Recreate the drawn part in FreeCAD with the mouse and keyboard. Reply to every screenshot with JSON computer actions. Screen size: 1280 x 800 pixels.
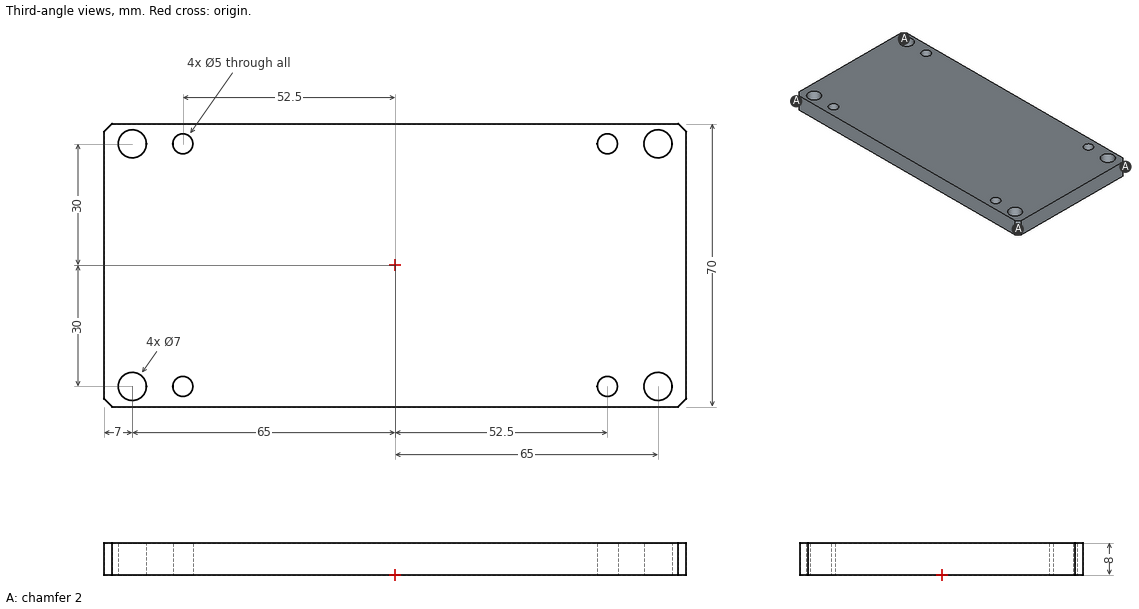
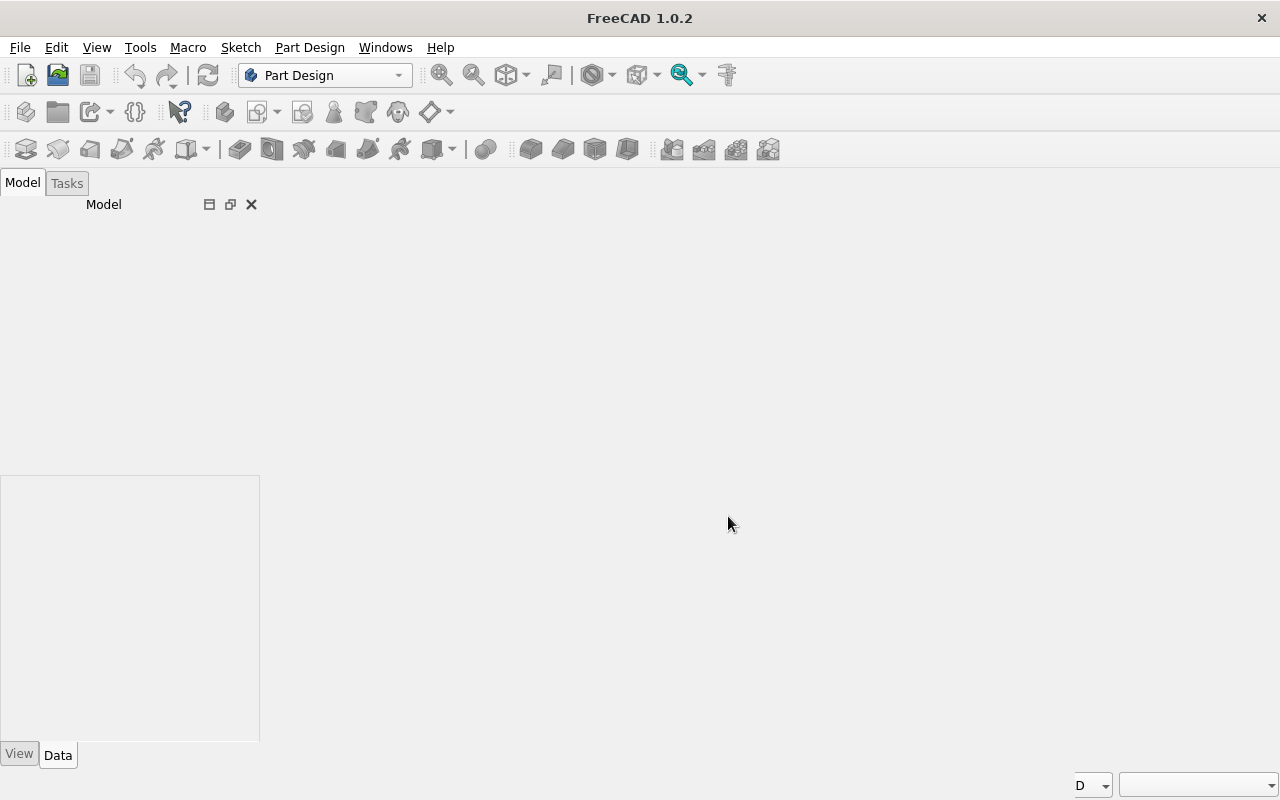
{"action": "left_click", "coordinate": [26, 76]}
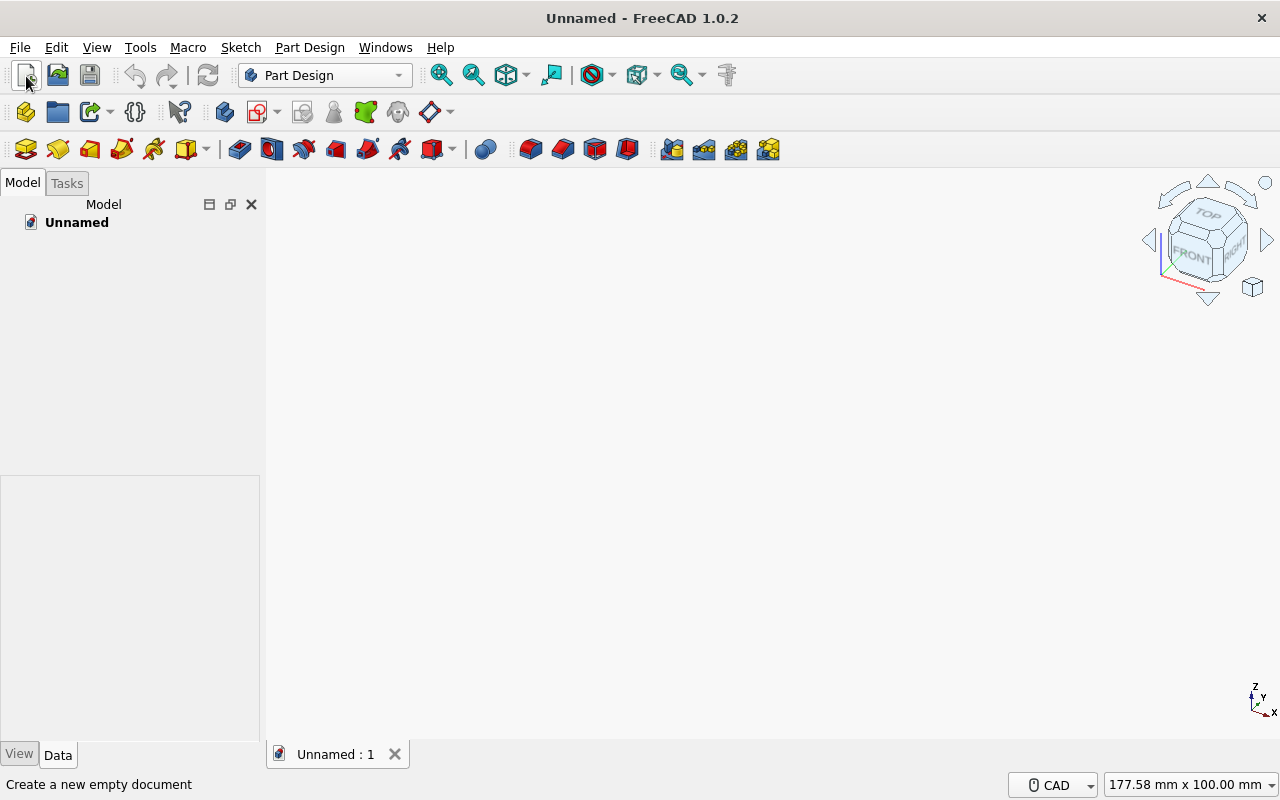
{"action": "left_click", "coordinate": [258, 112]}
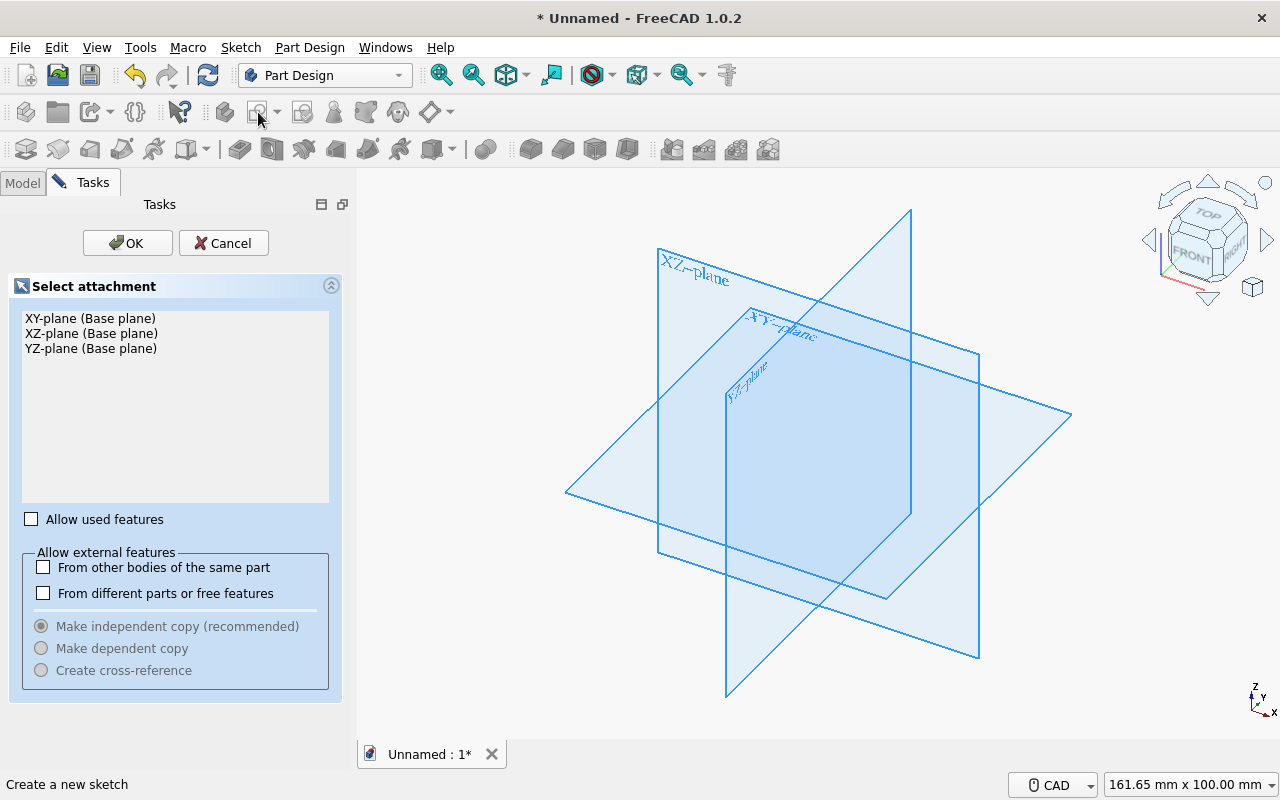
{"action": "left_click", "coordinate": [82, 318]}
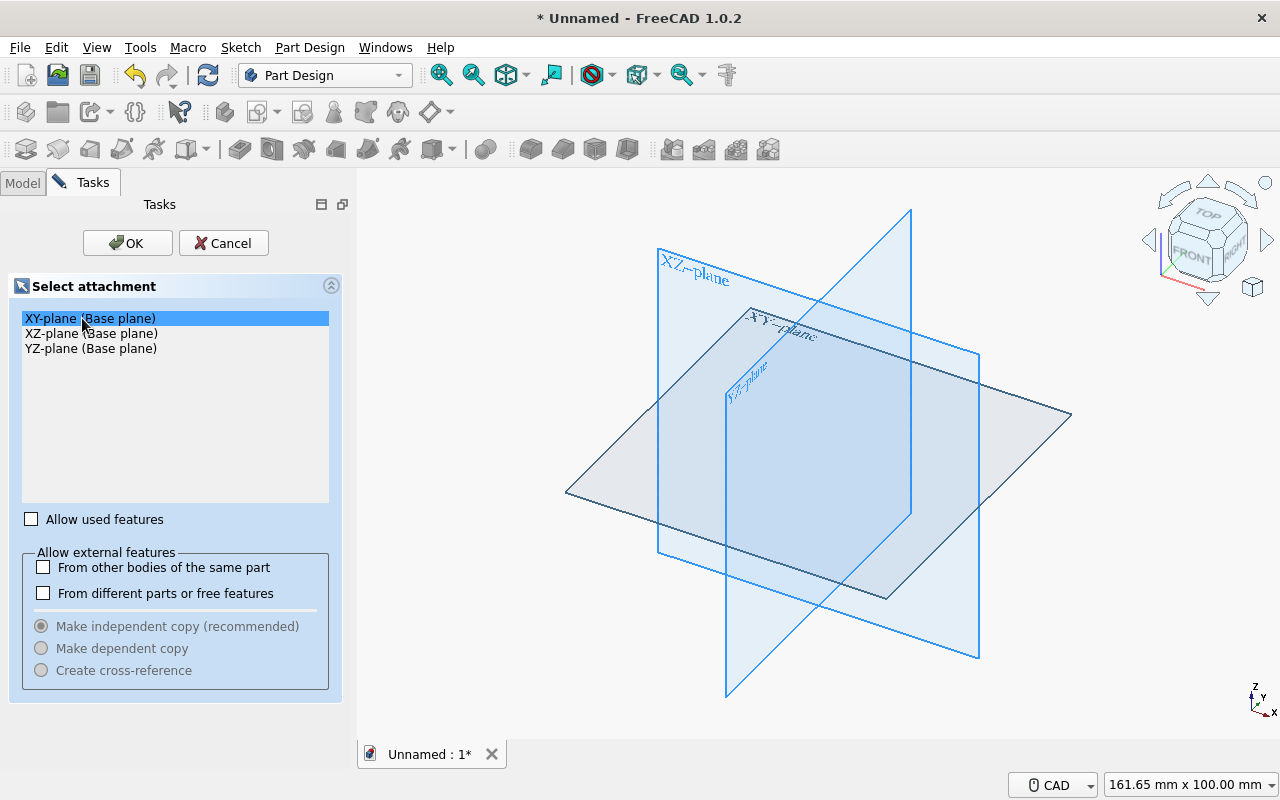
{"action": "left_click", "coordinate": [128, 243]}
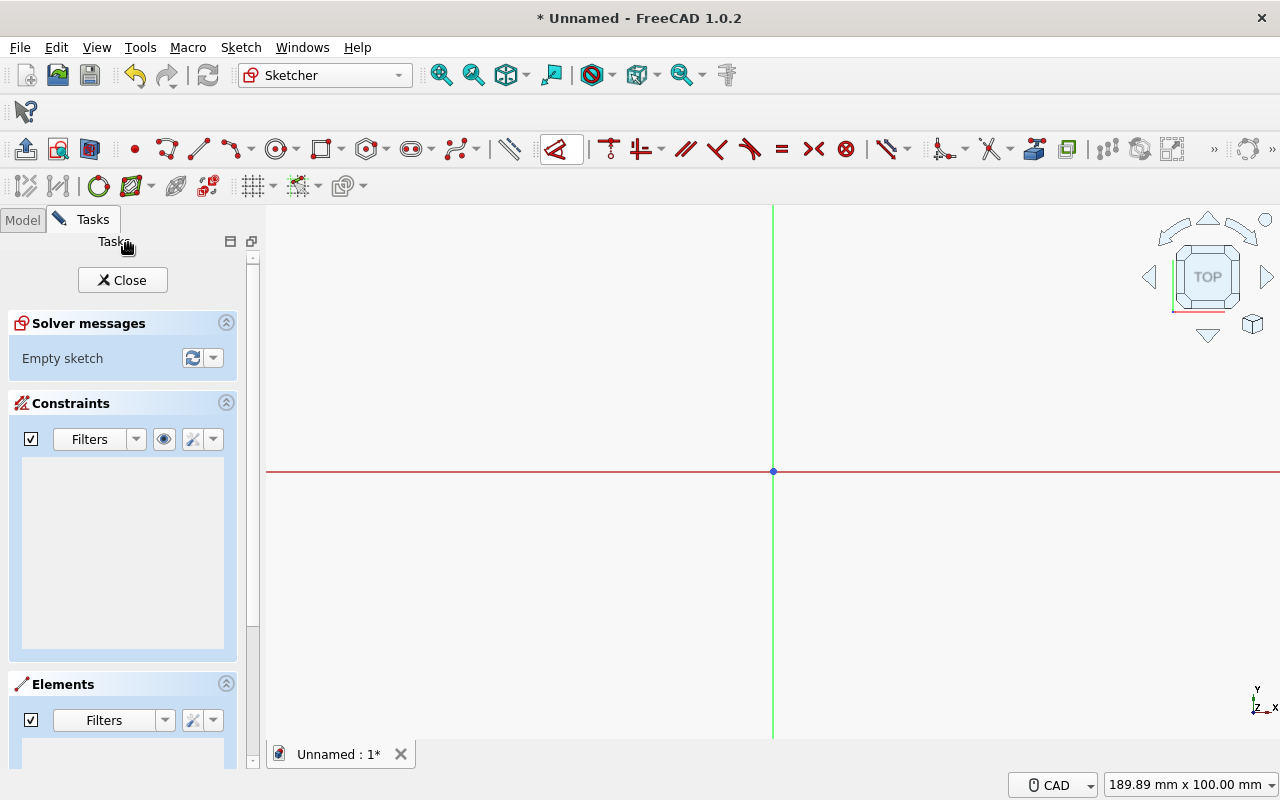
{"action": "scroll", "coordinate": [395, 472], "scroll_direction": "down", "scroll_amount": 1}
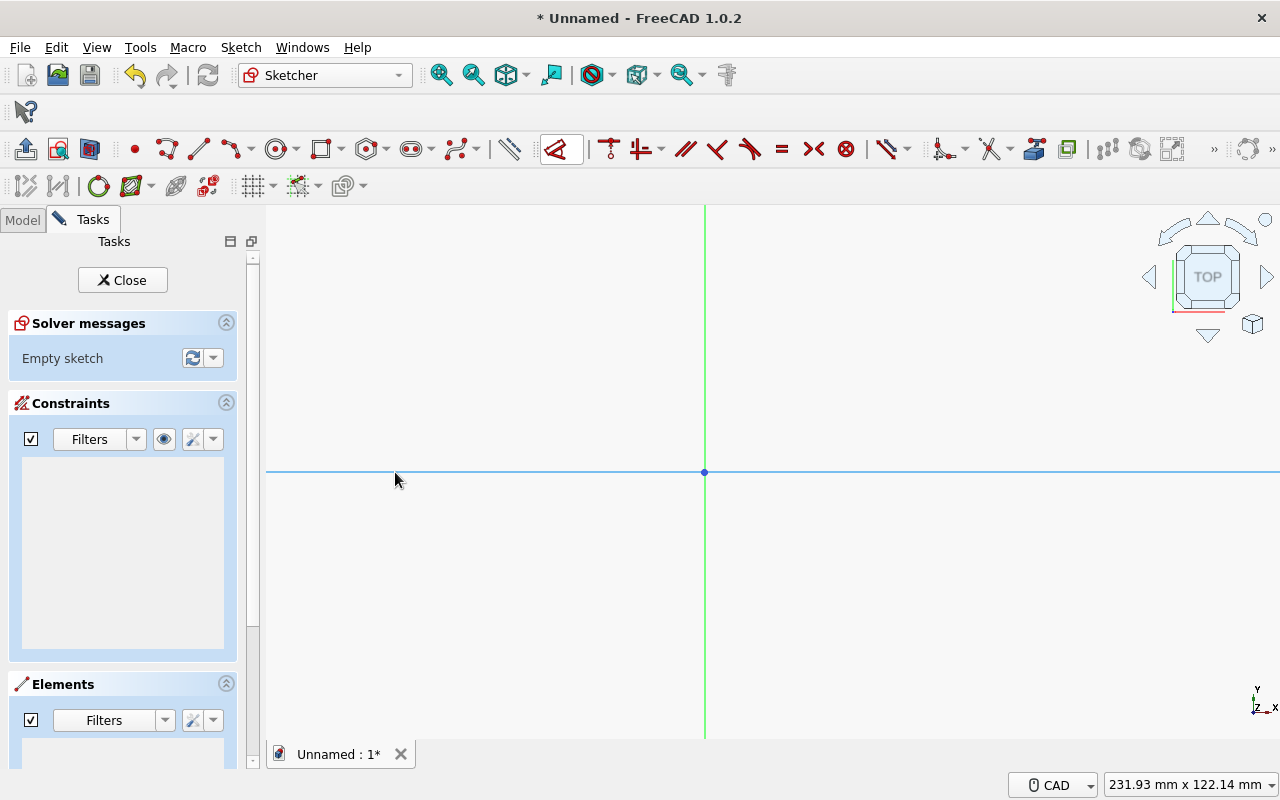
{"action": "key", "text": "g v"}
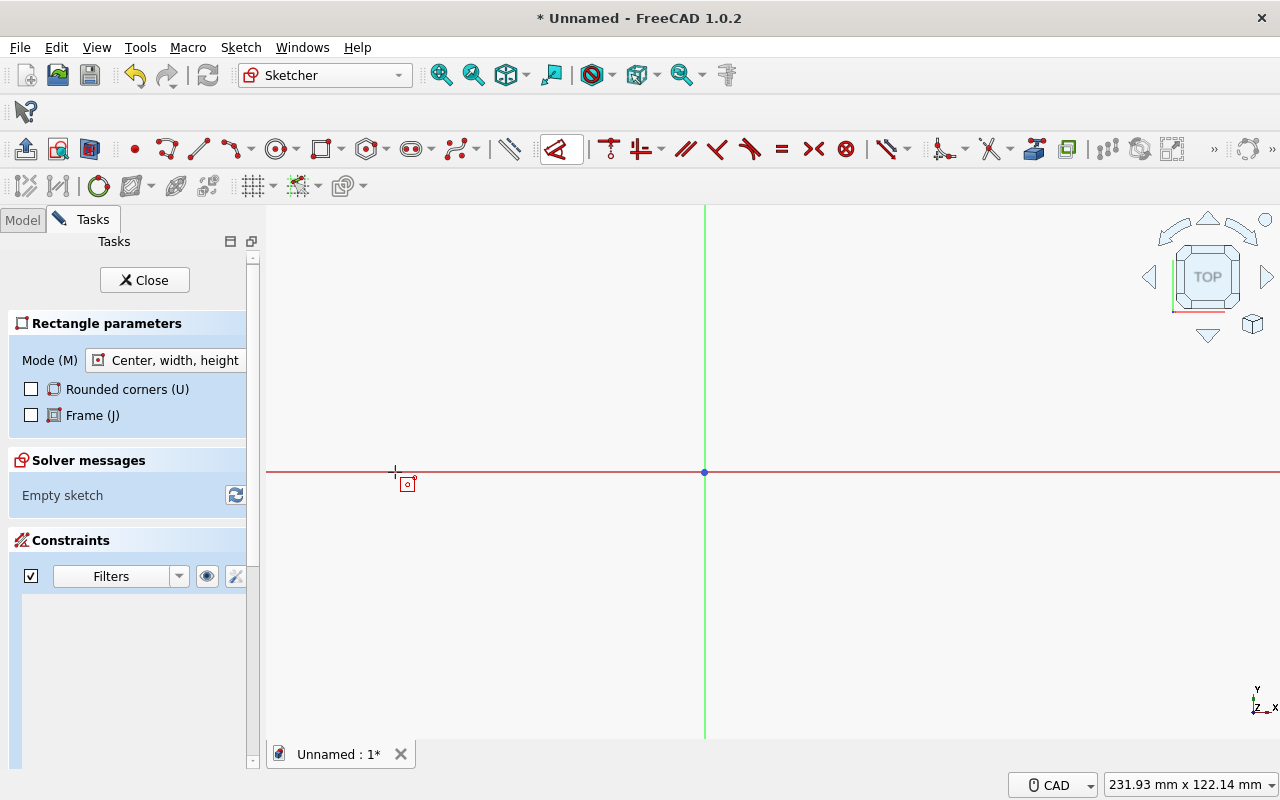
{"action": "left_click", "coordinate": [705, 472]}
{"action": "left_click", "coordinate": [1019, 319]}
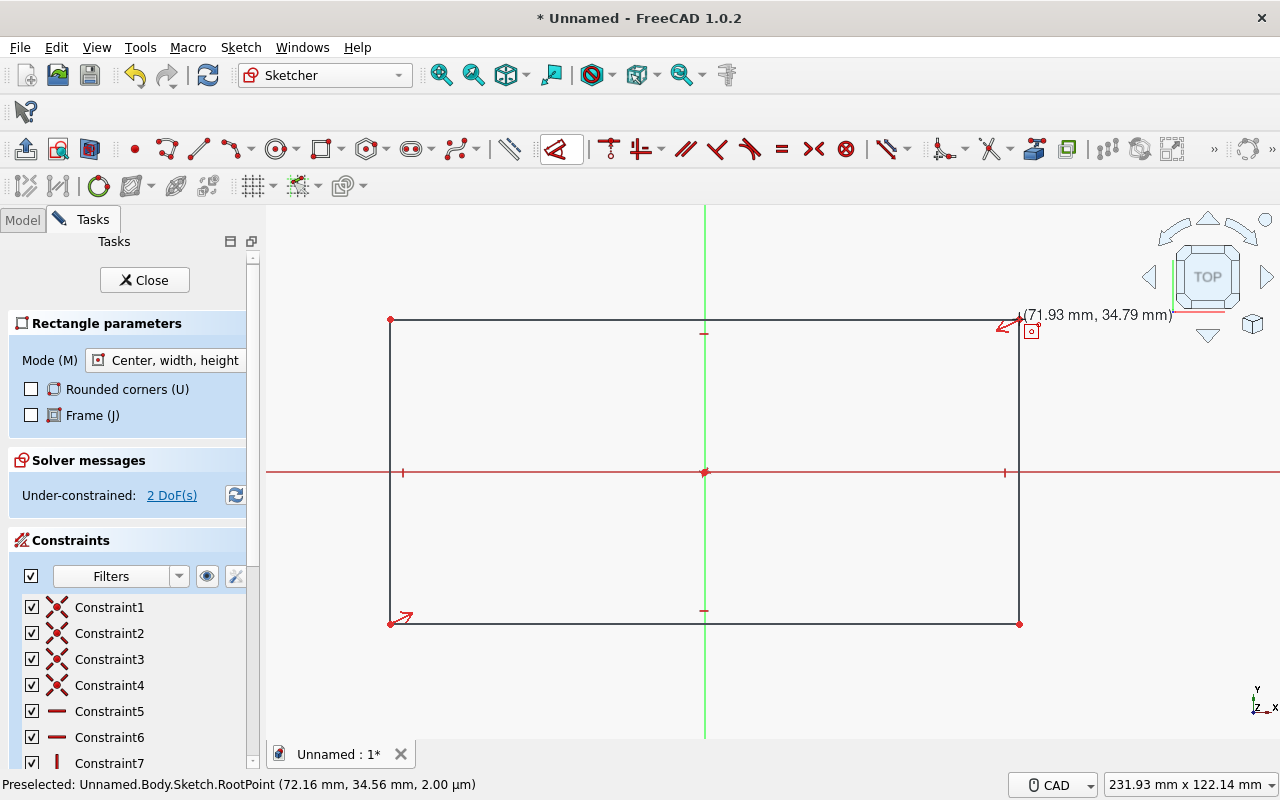
{"action": "left_click", "coordinate": [276, 150]}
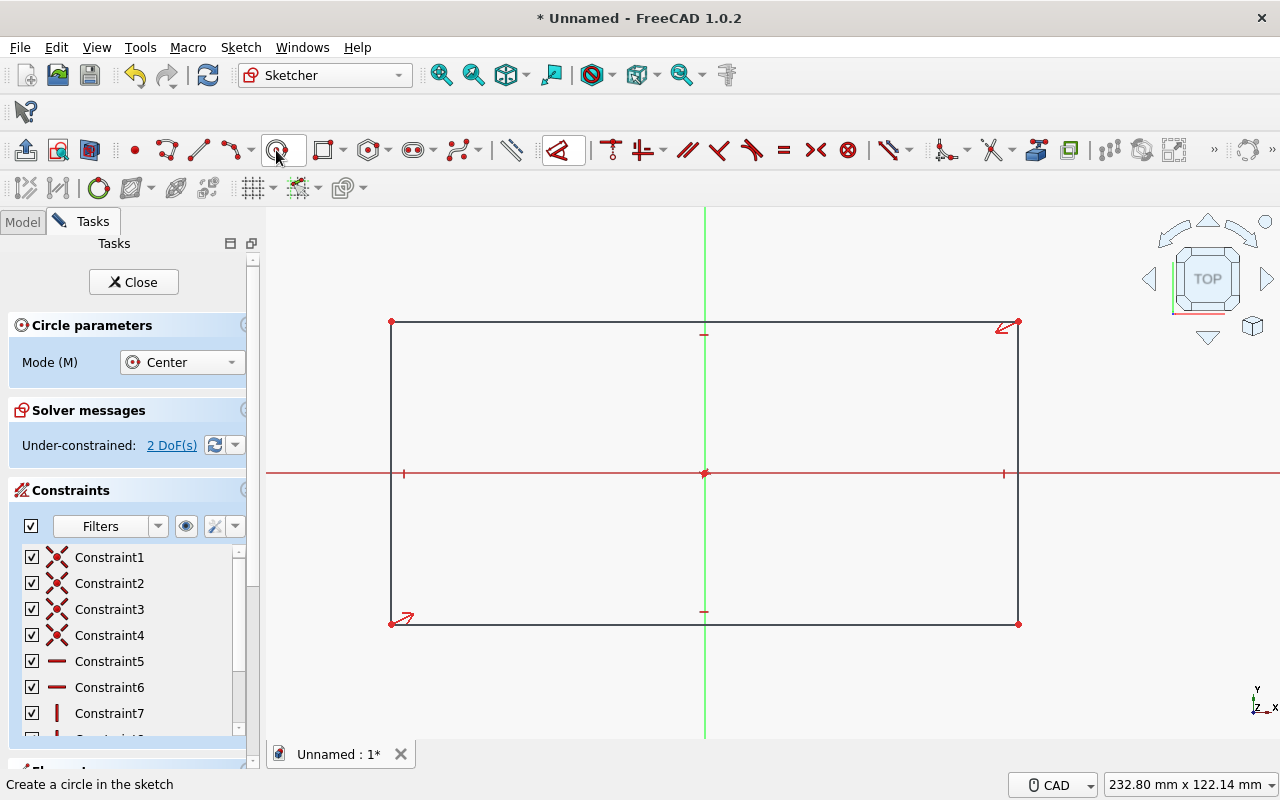
{"action": "scroll", "coordinate": [422, 604], "scroll_direction": "up", "scroll_amount": 2}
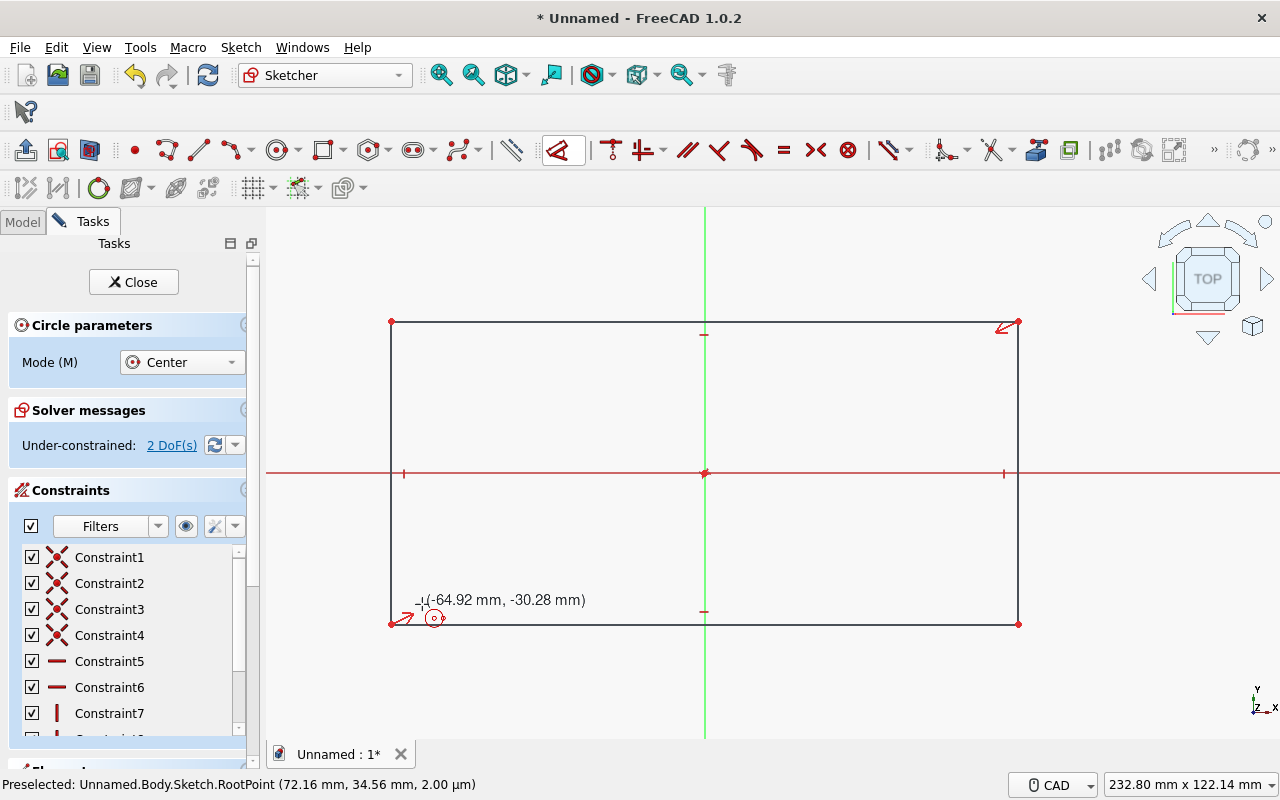
{"action": "left_click", "coordinate": [421, 603]}
{"action": "left_click", "coordinate": [437, 587]}